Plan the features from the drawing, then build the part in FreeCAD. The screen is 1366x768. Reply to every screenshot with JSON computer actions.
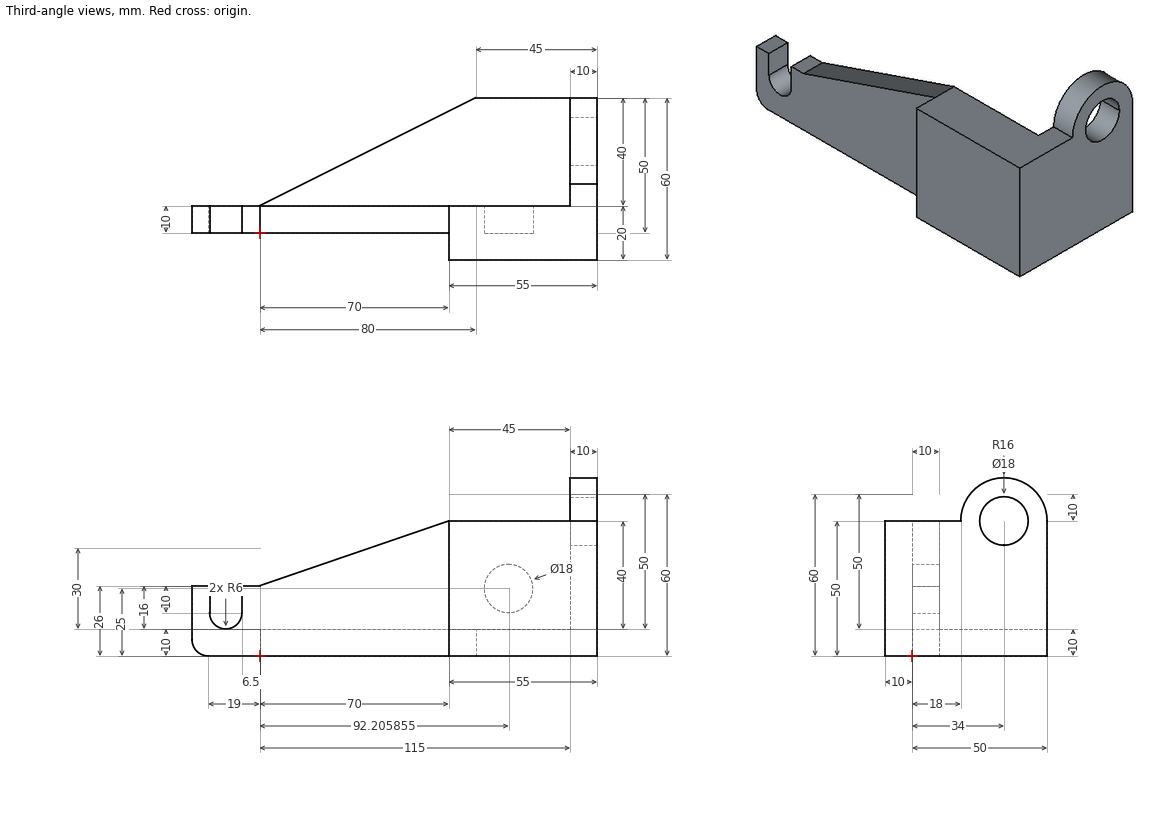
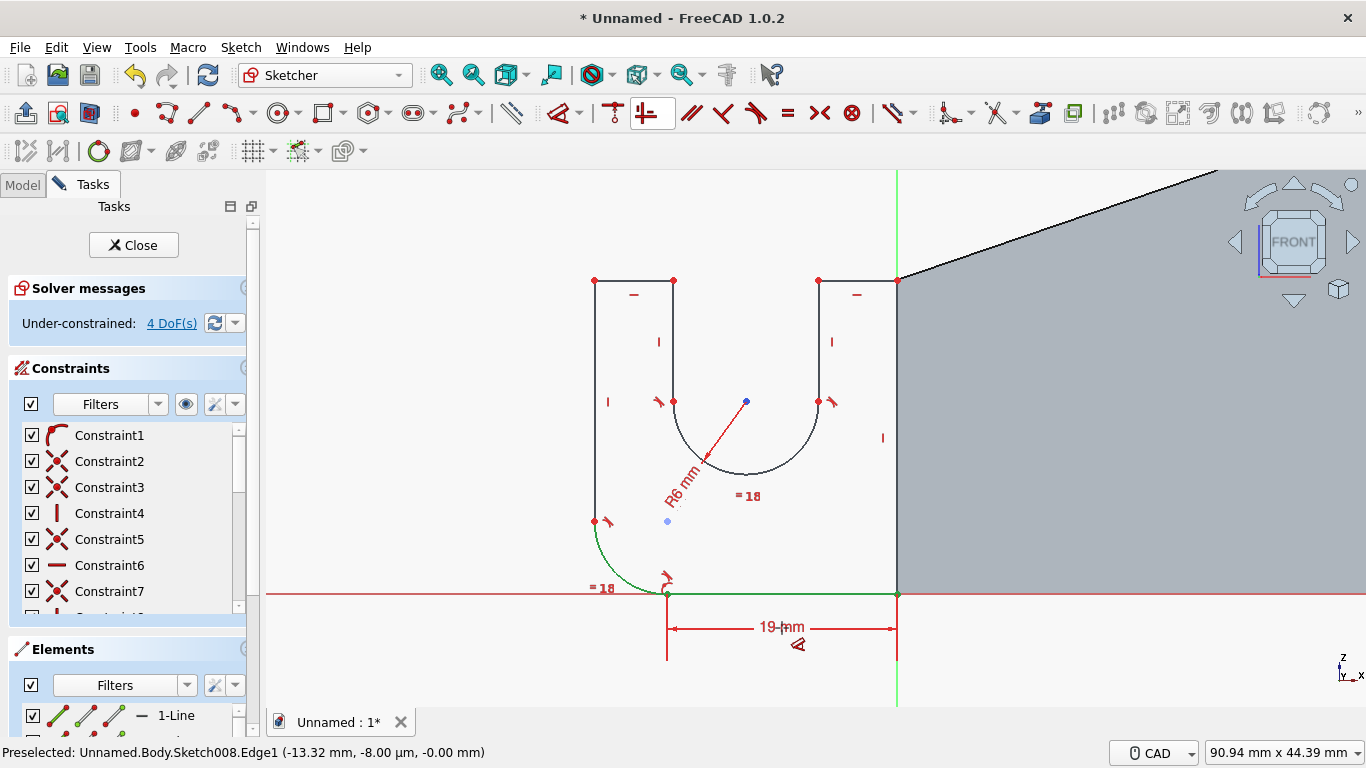
{"action": "left_click", "coordinate": [897, 500]}
{"action": "left_click", "coordinate": [931, 438]}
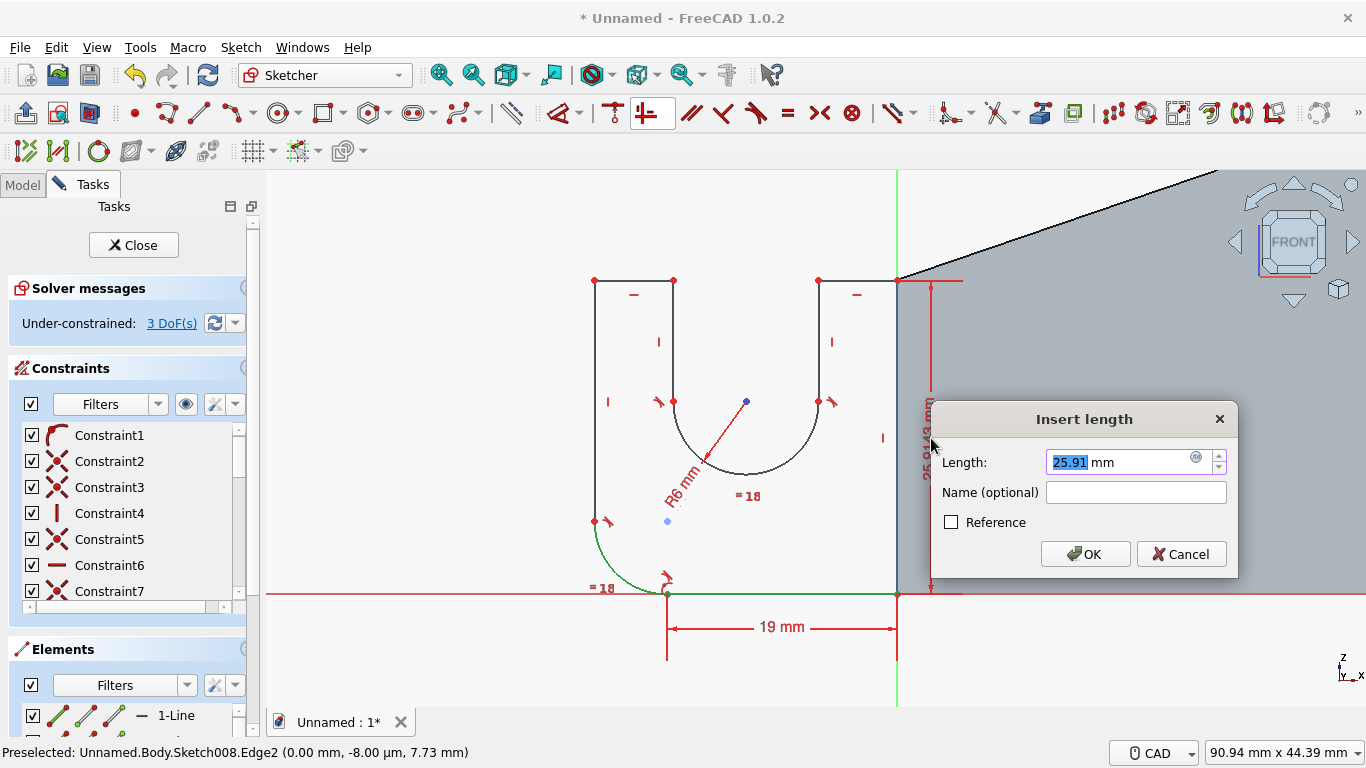
{"action": "type", "text": "26"}
{"action": "key", "text": "Return"}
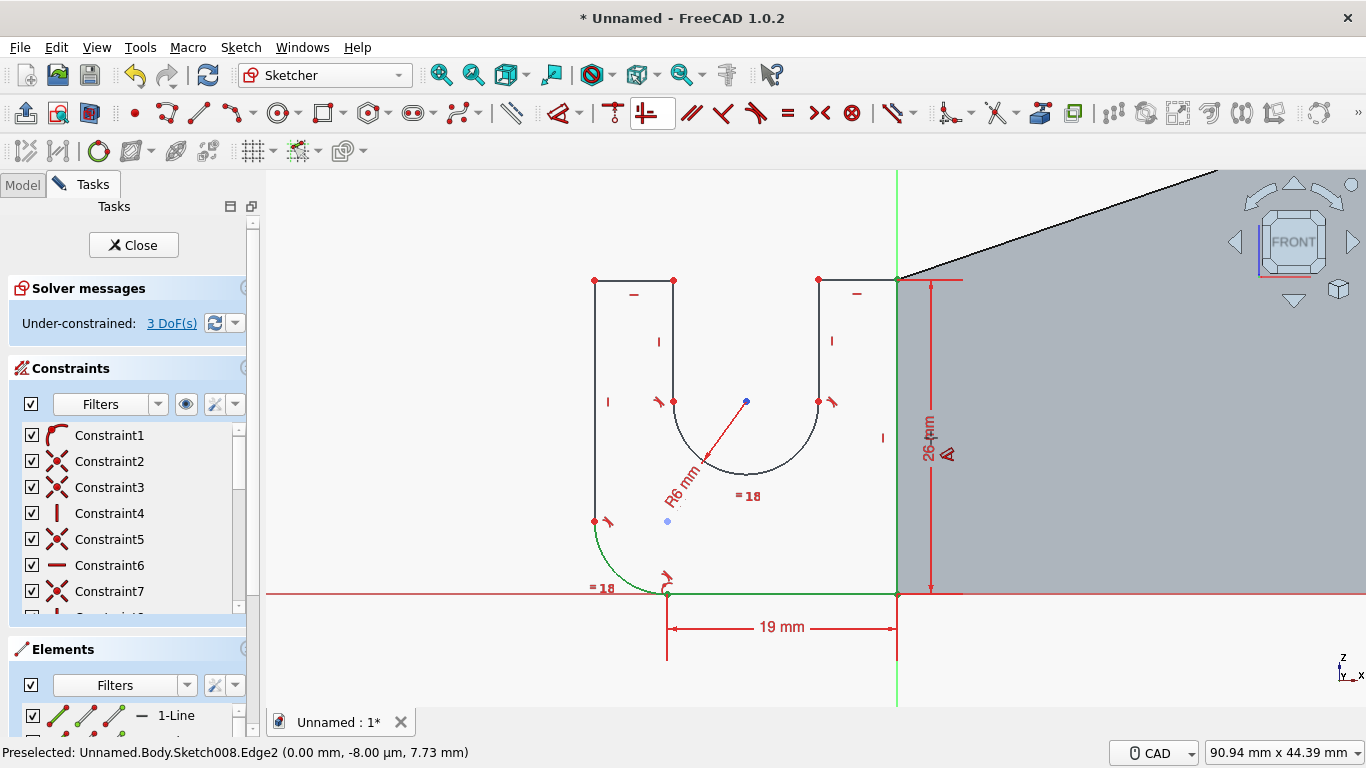
{"action": "left_click", "coordinate": [819, 317]}
{"action": "left_click", "coordinate": [853, 341]}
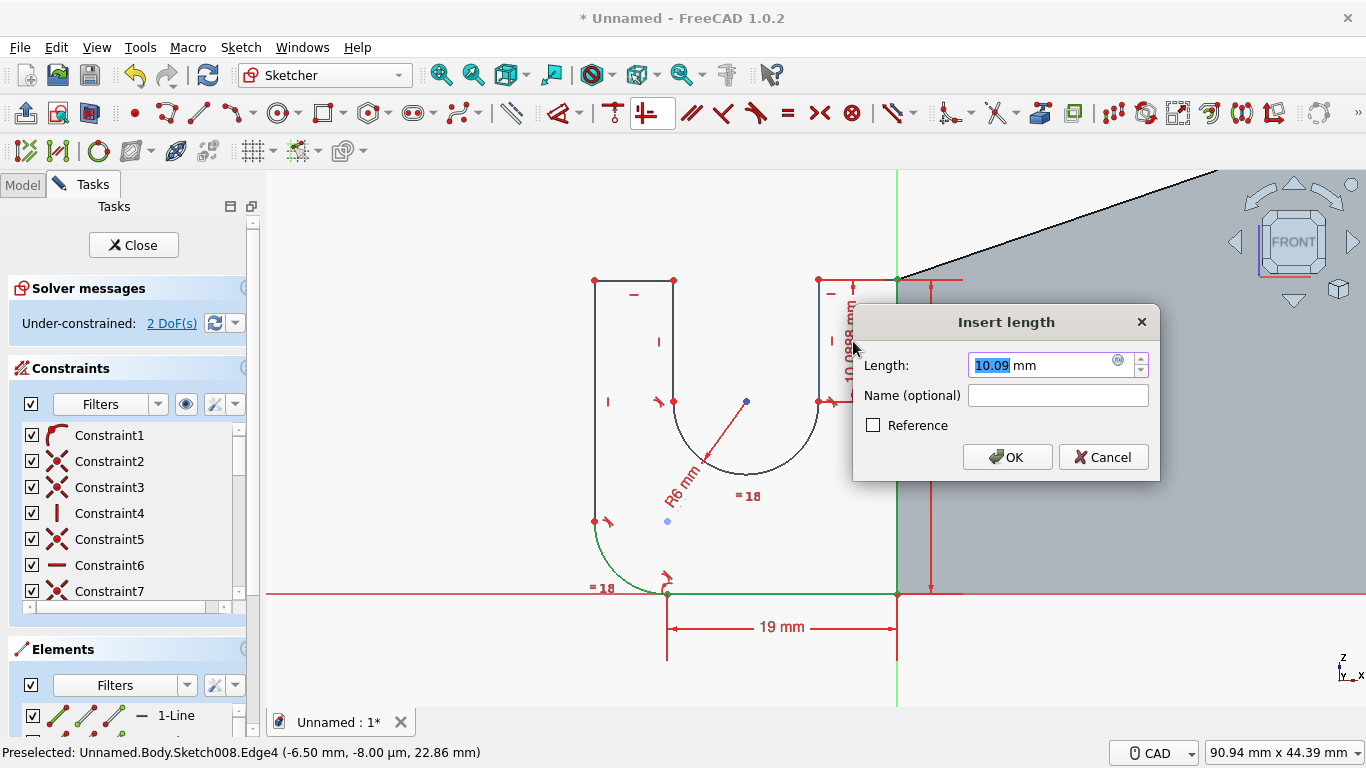
{"action": "type", "text": "10"}
{"action": "key", "text": "Return"}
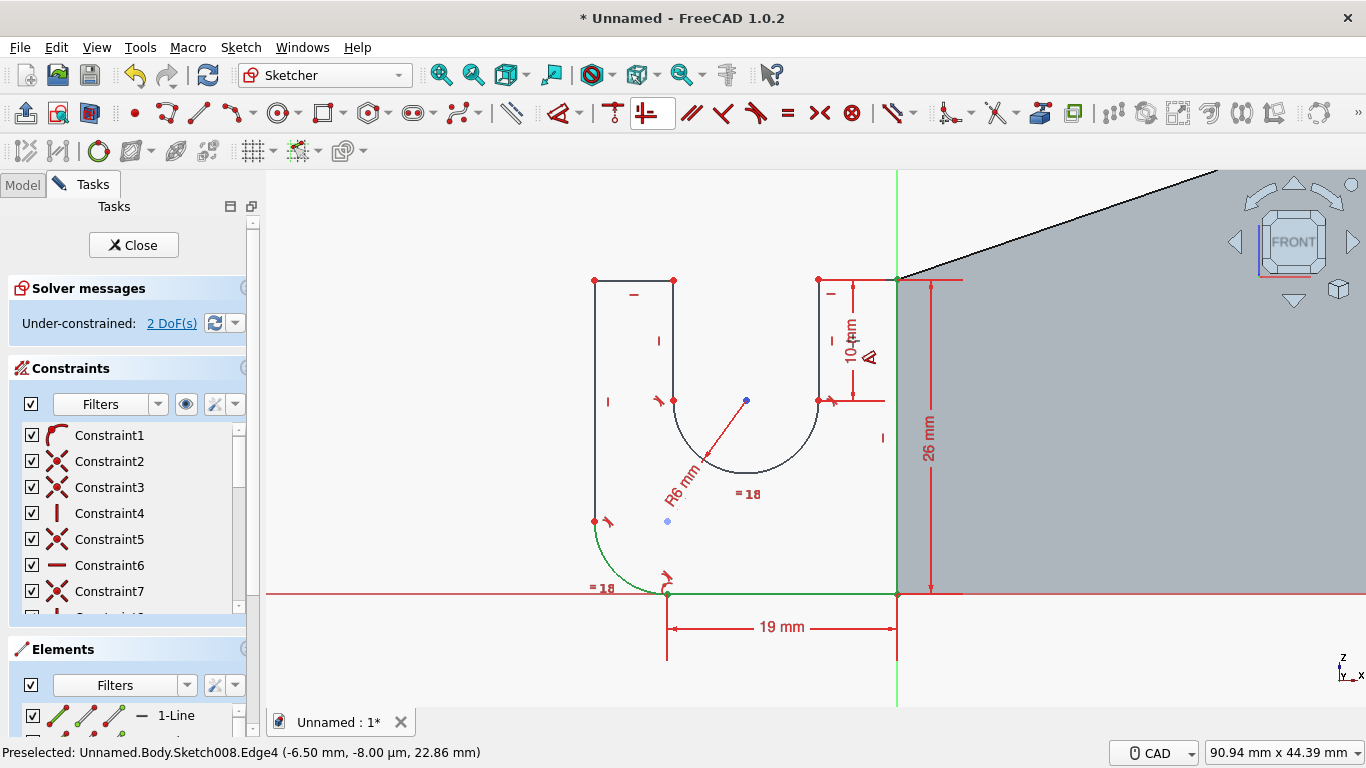
{"action": "left_click", "coordinate": [673, 365]}
{"action": "left_click", "coordinate": [639, 341]}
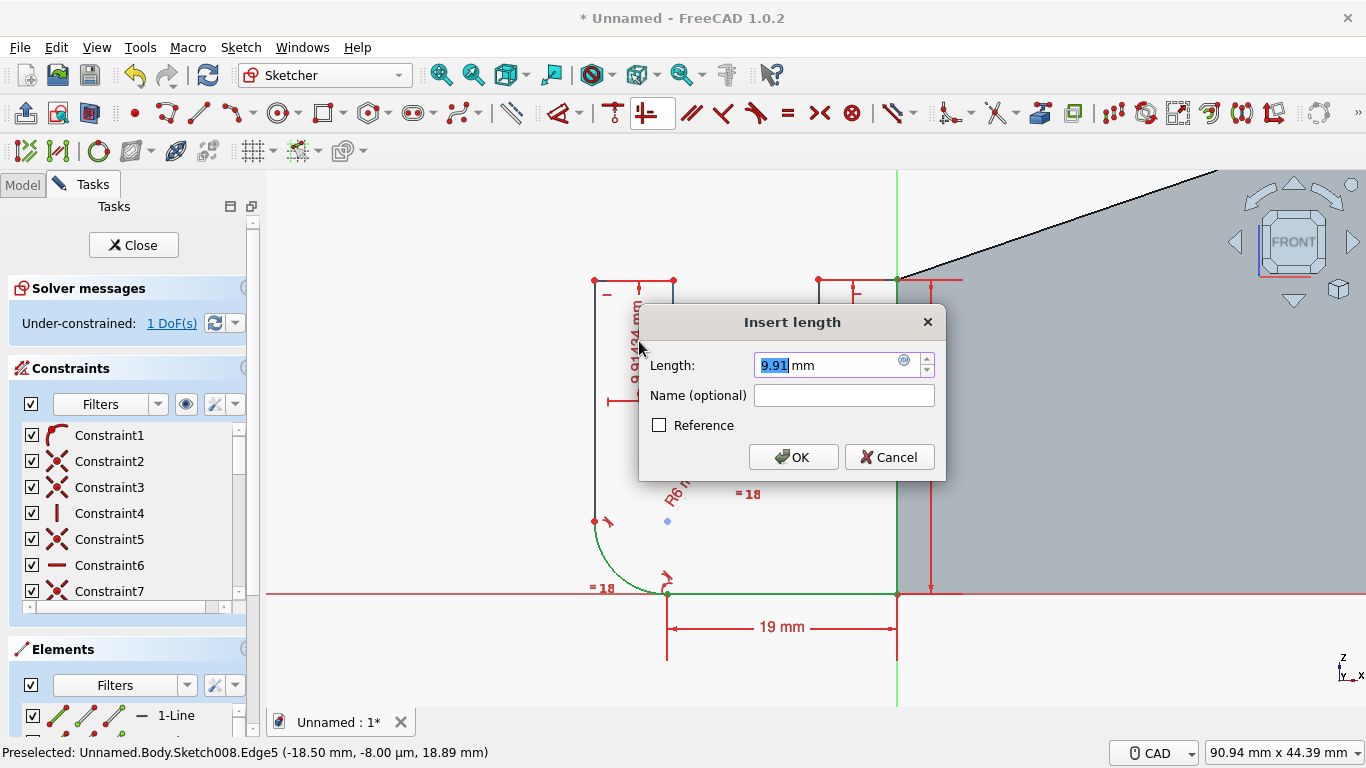
{"action": "type", "text": "10"}
{"action": "key", "text": "Return"}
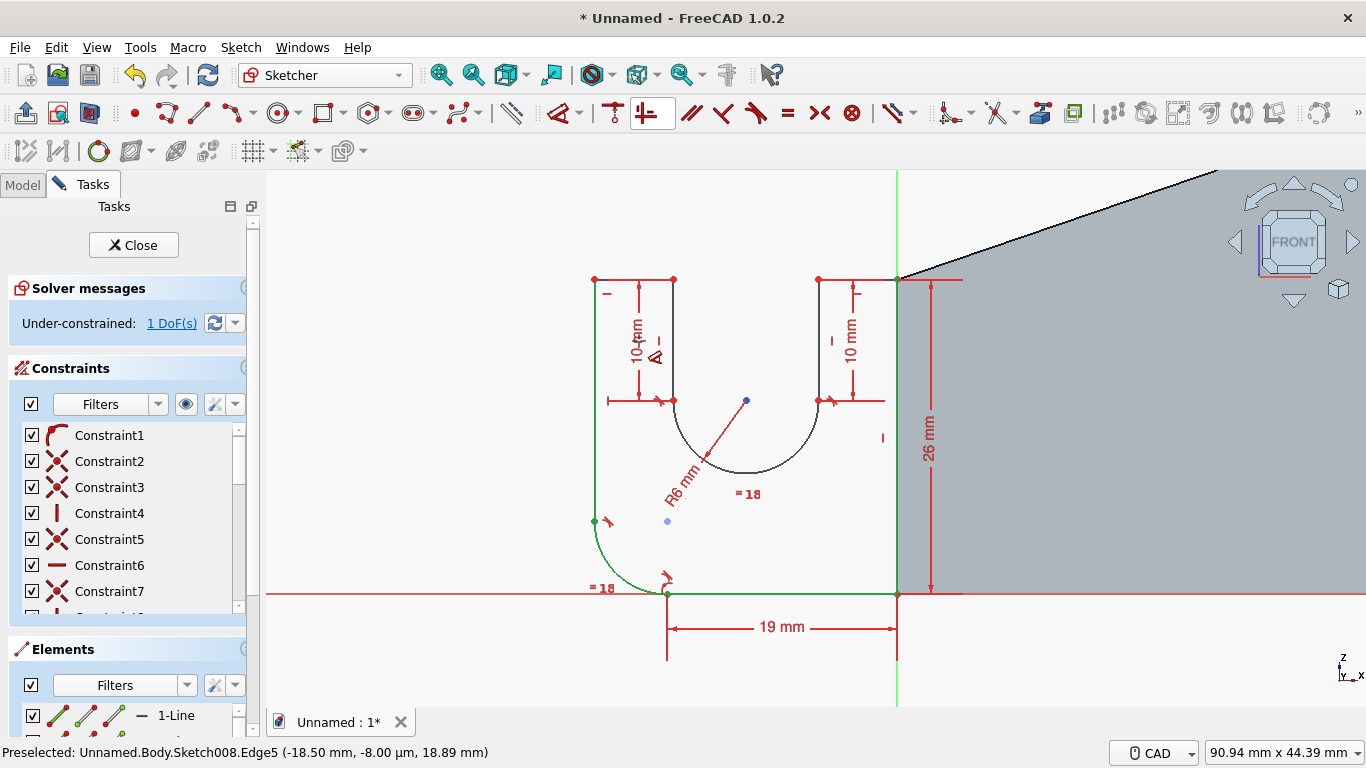
{"action": "left_click", "coordinate": [874, 280]}
{"action": "left_click", "coordinate": [858, 246]}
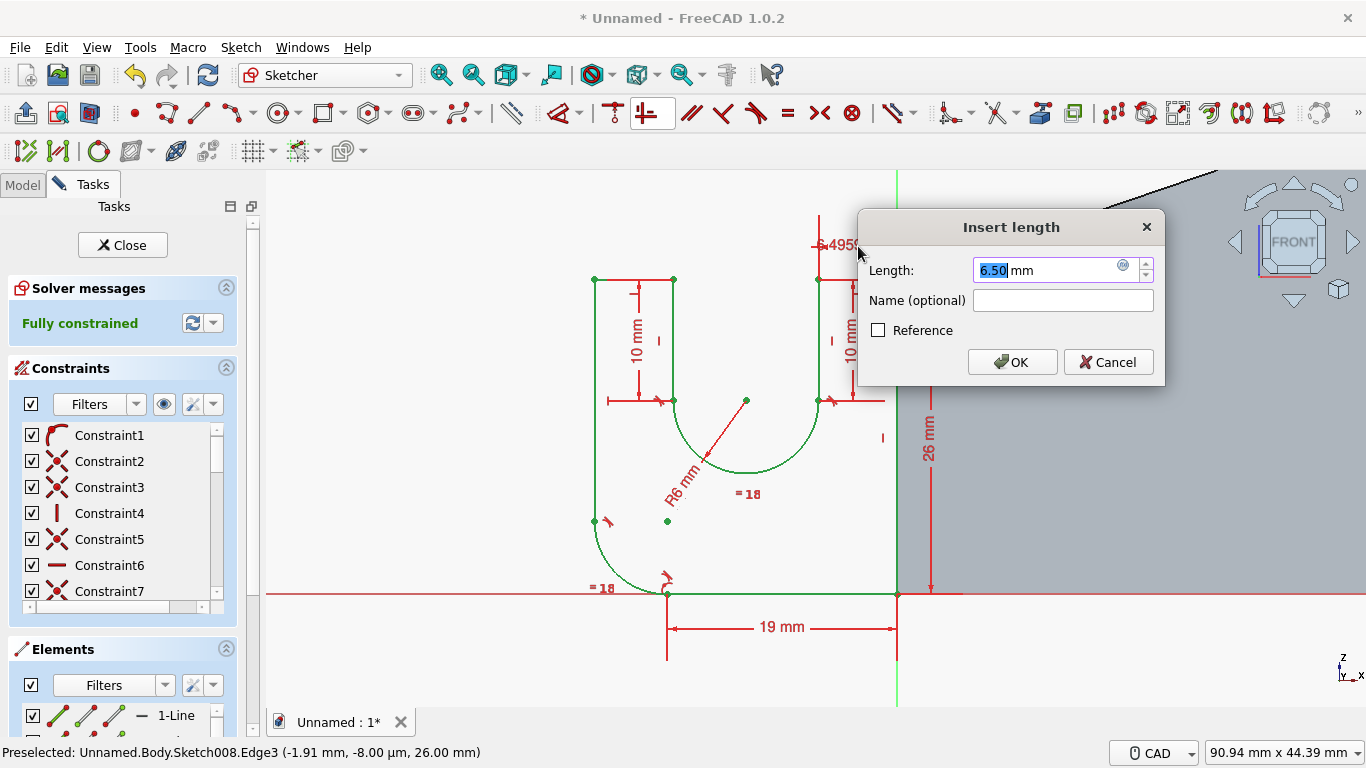
{"action": "type", "text": "6.5"}
{"action": "key", "text": "Return"}
{"action": "key", "text": "Escape"}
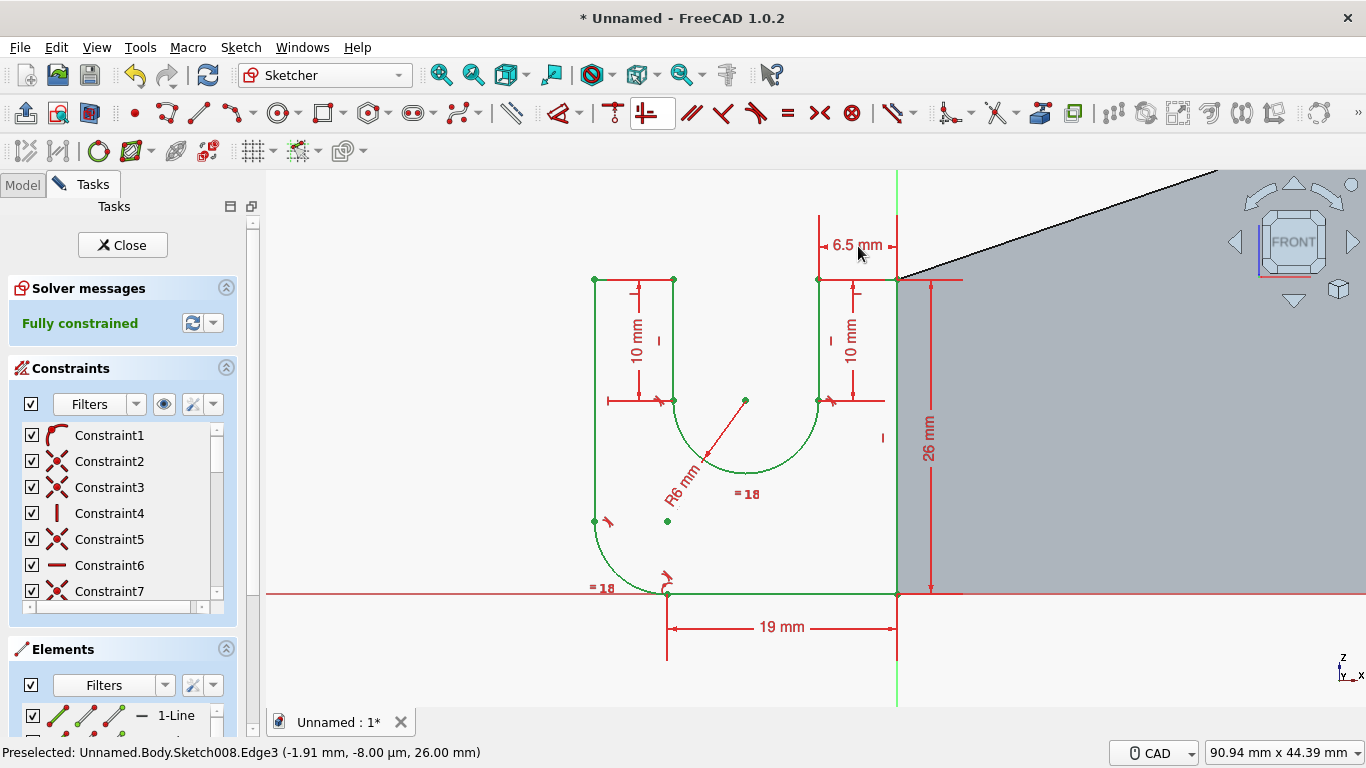
{"action": "left_click", "coordinate": [123, 245]}